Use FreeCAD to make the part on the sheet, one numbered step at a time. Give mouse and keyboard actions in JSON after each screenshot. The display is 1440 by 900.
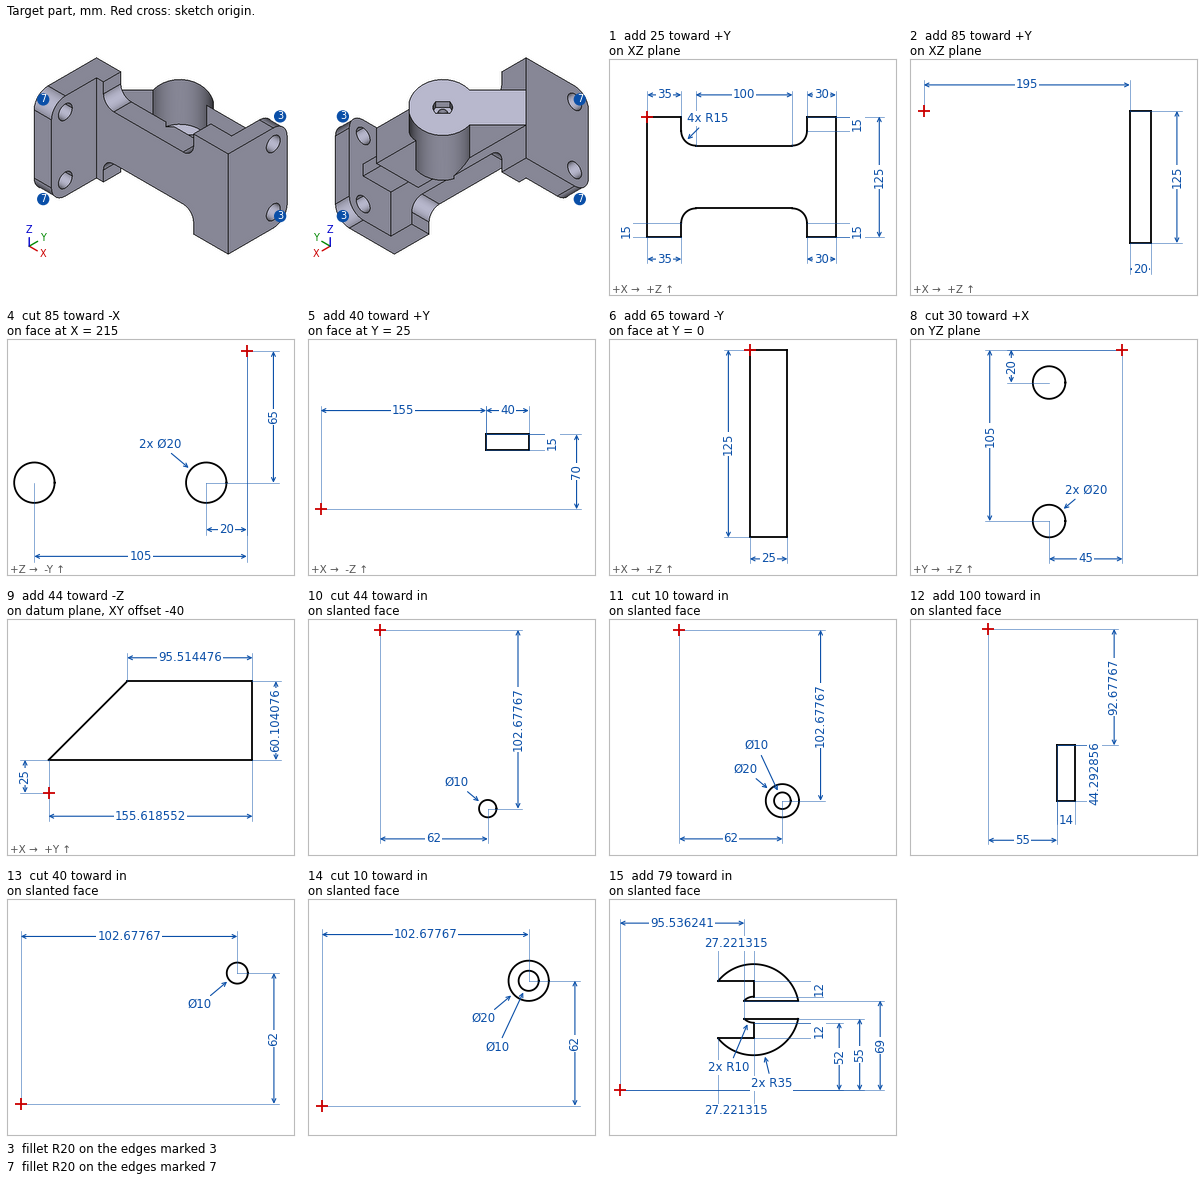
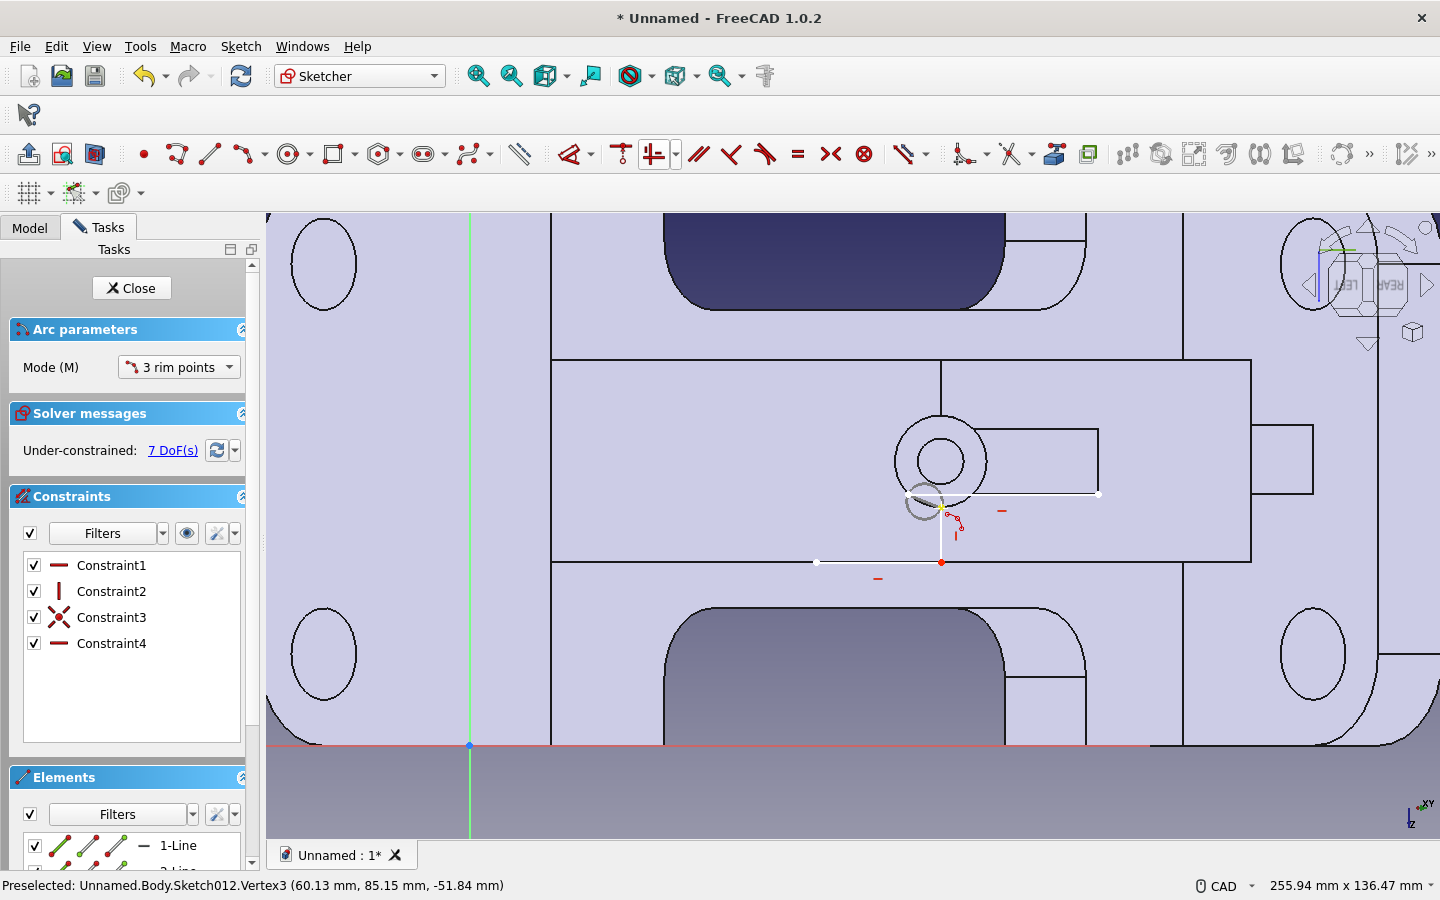
{"action": "scroll", "coordinate": [923, 504], "scroll_direction": "up", "scroll_amount": 8}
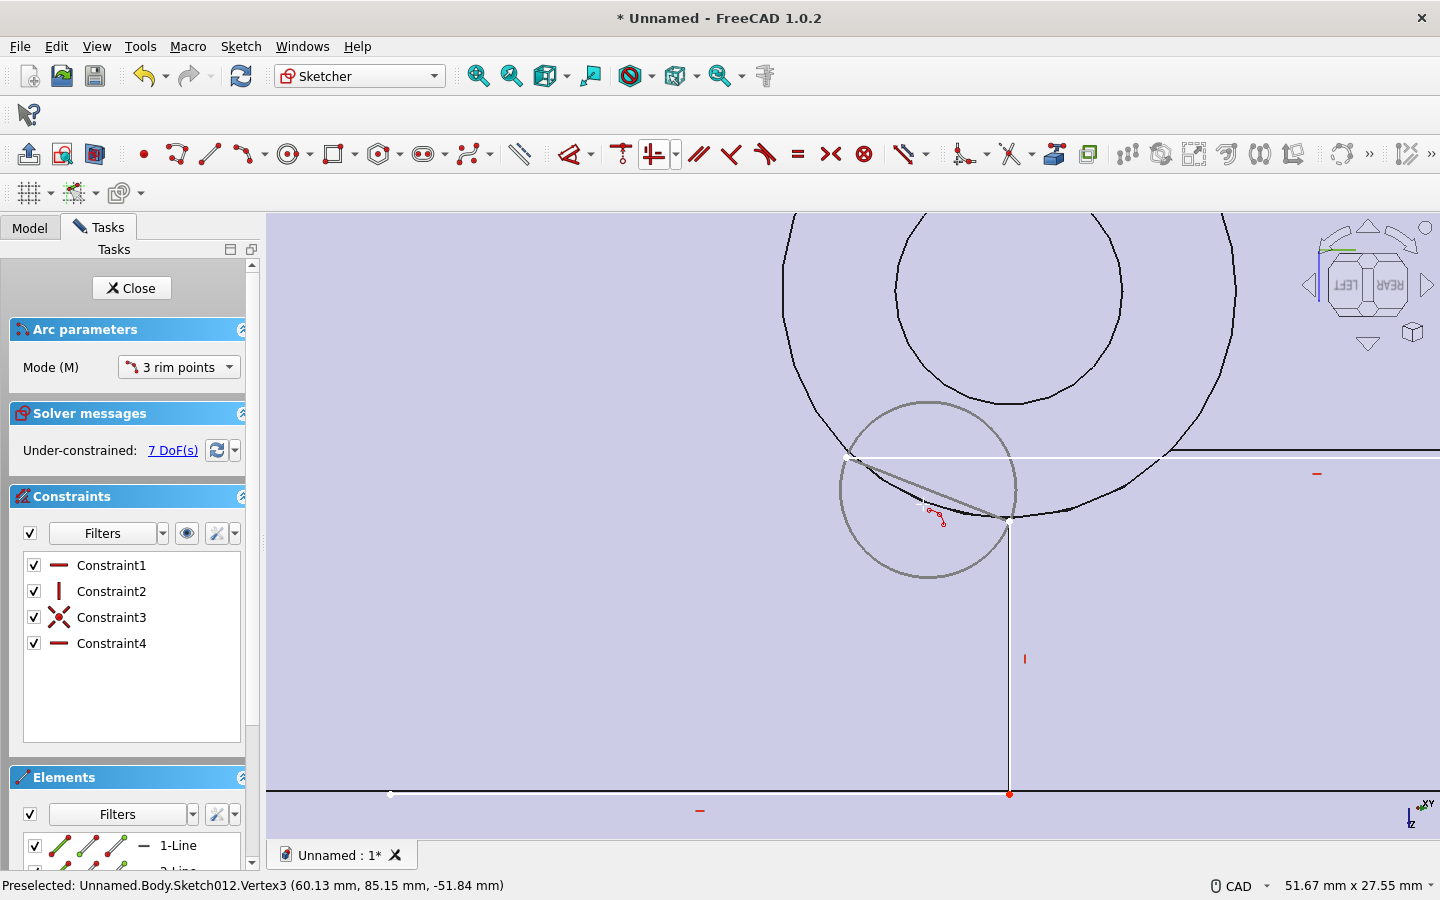
{"action": "left_click", "coordinate": [921, 501]}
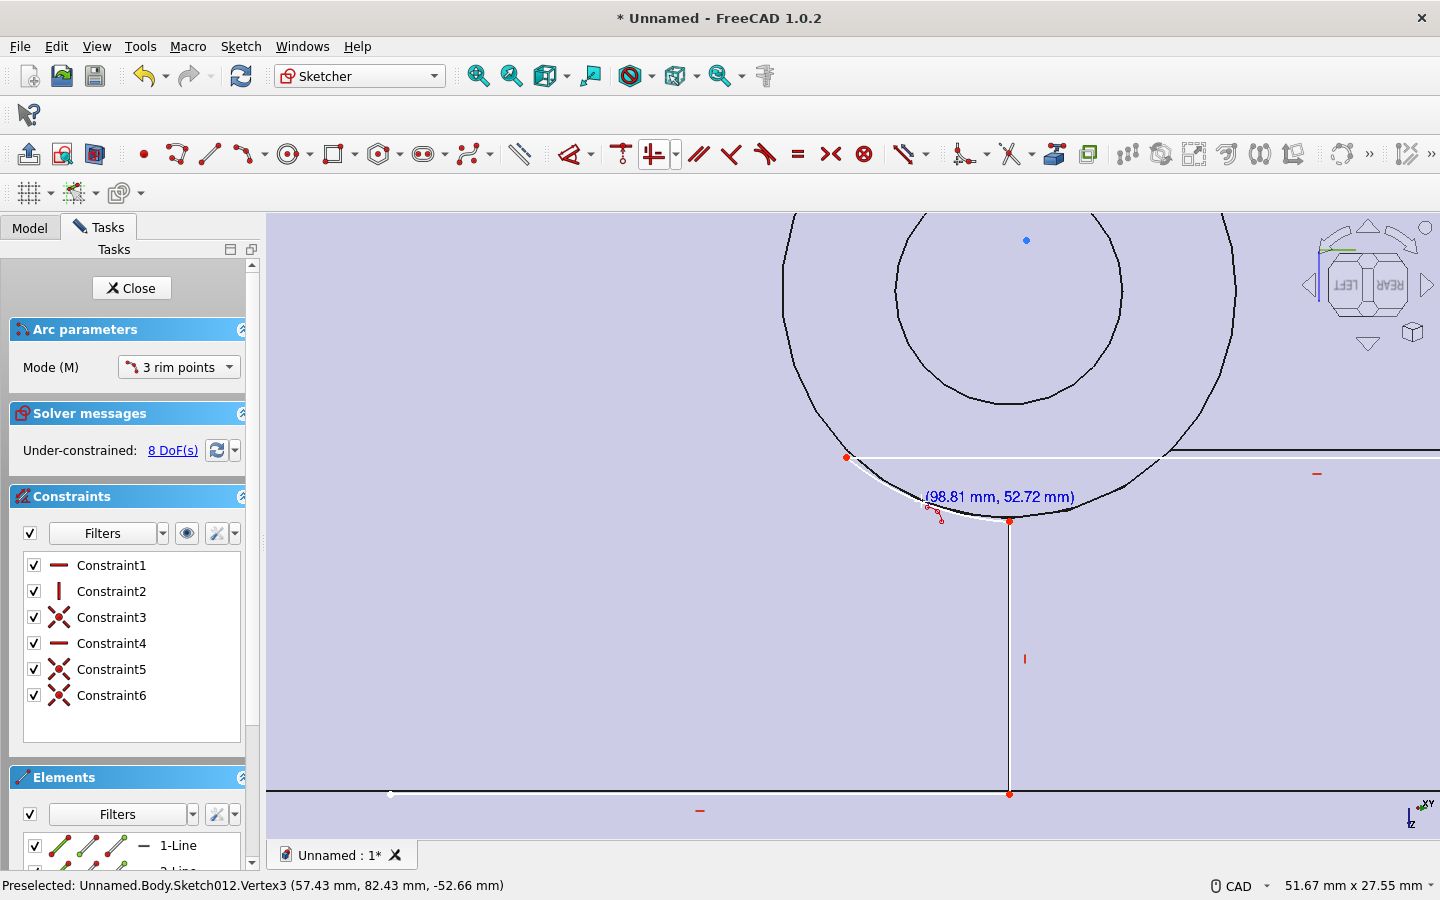
{"action": "scroll", "coordinate": [924, 505], "scroll_direction": "down", "scroll_amount": 8}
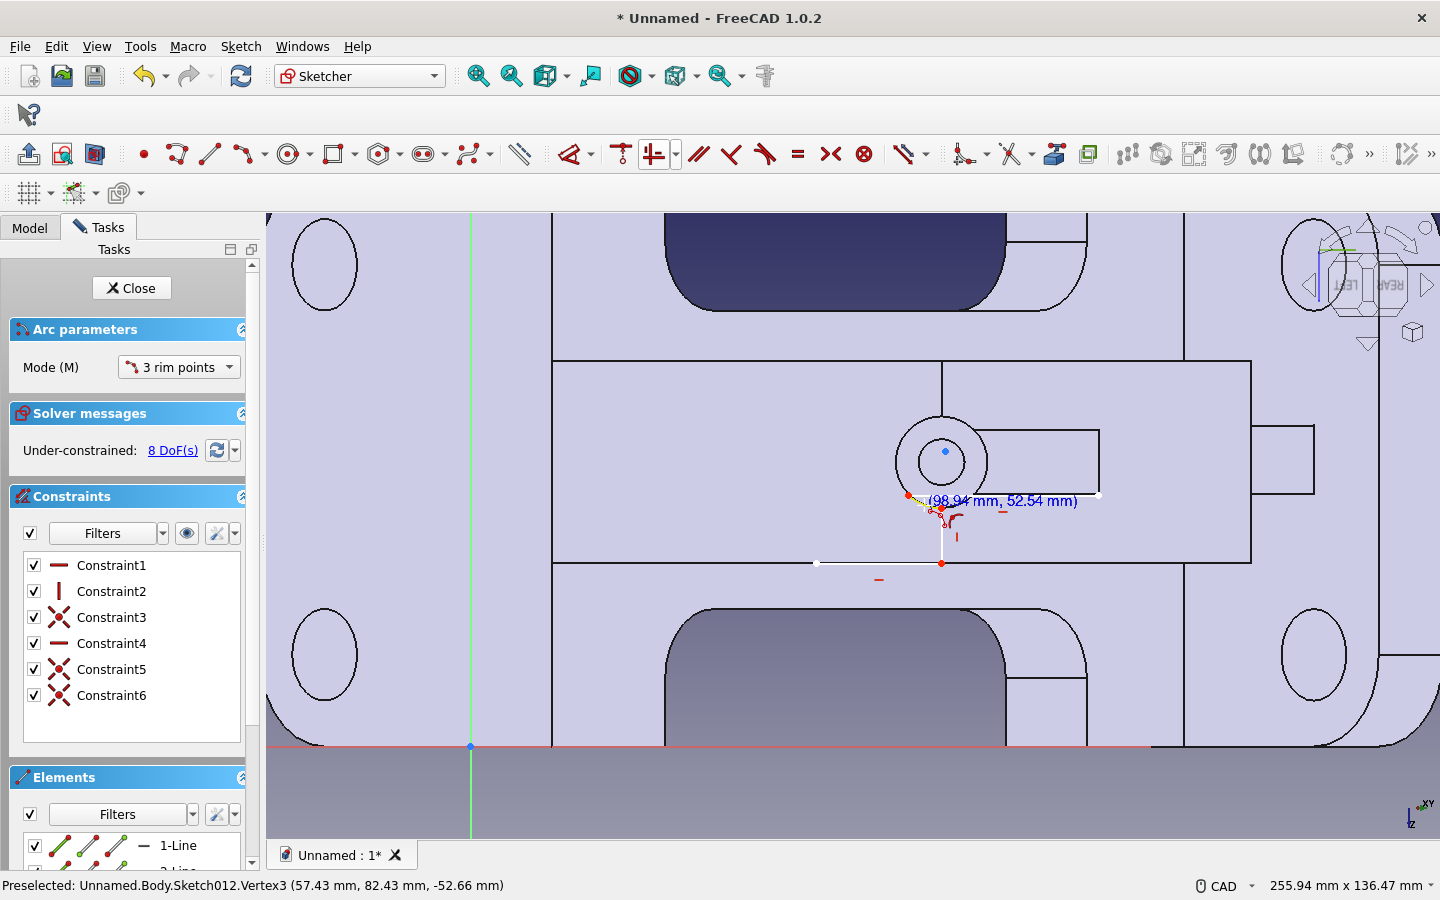
{"action": "left_click", "coordinate": [817, 564]}
{"action": "left_click", "coordinate": [1099, 496]}
{"action": "left_click", "coordinate": [980, 618]}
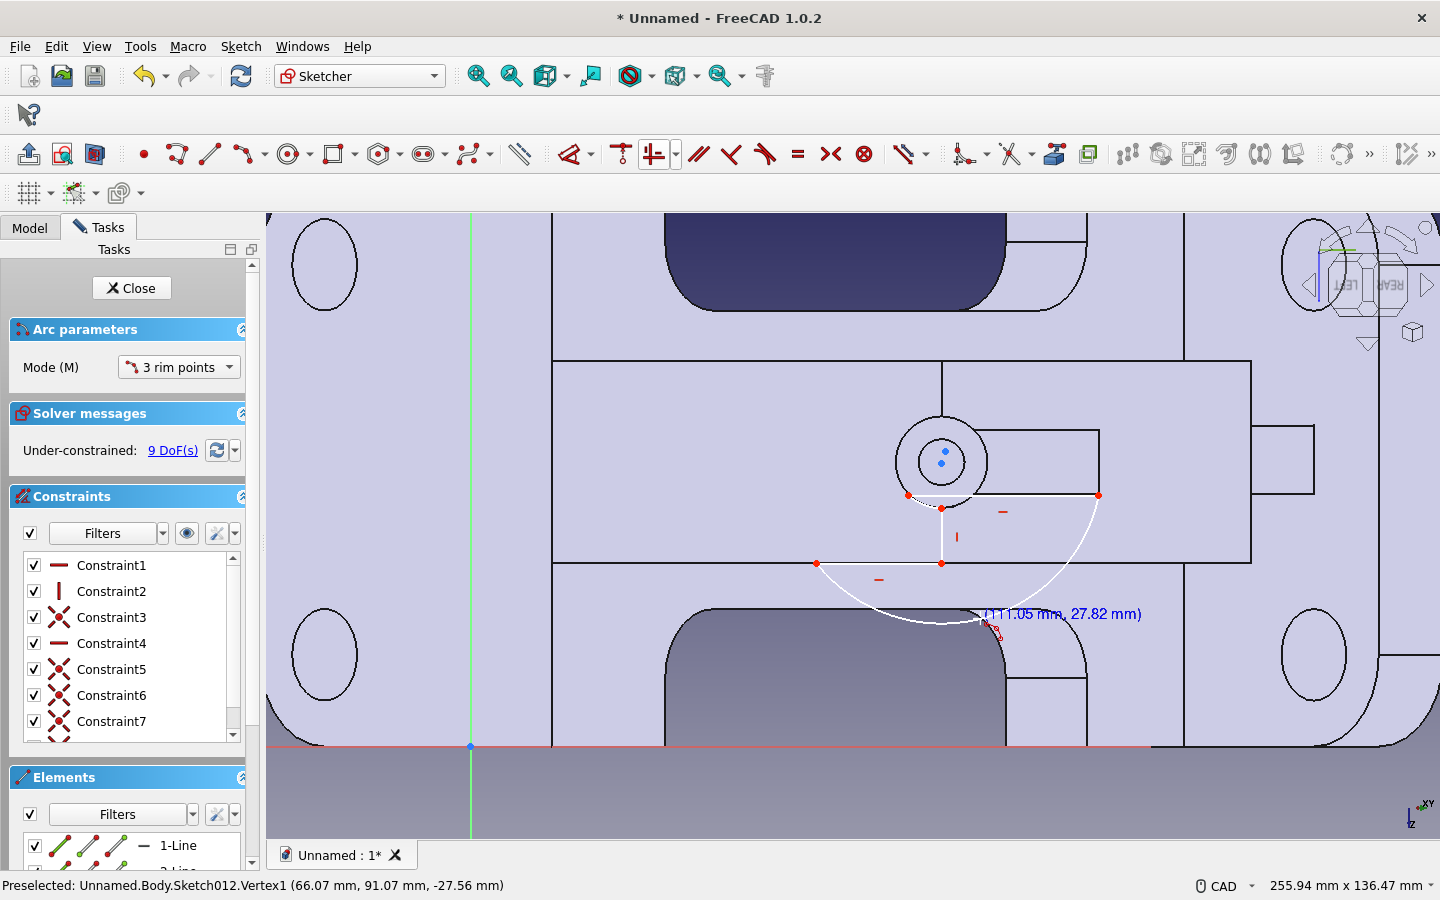
{"action": "left_click", "coordinate": [210, 154]}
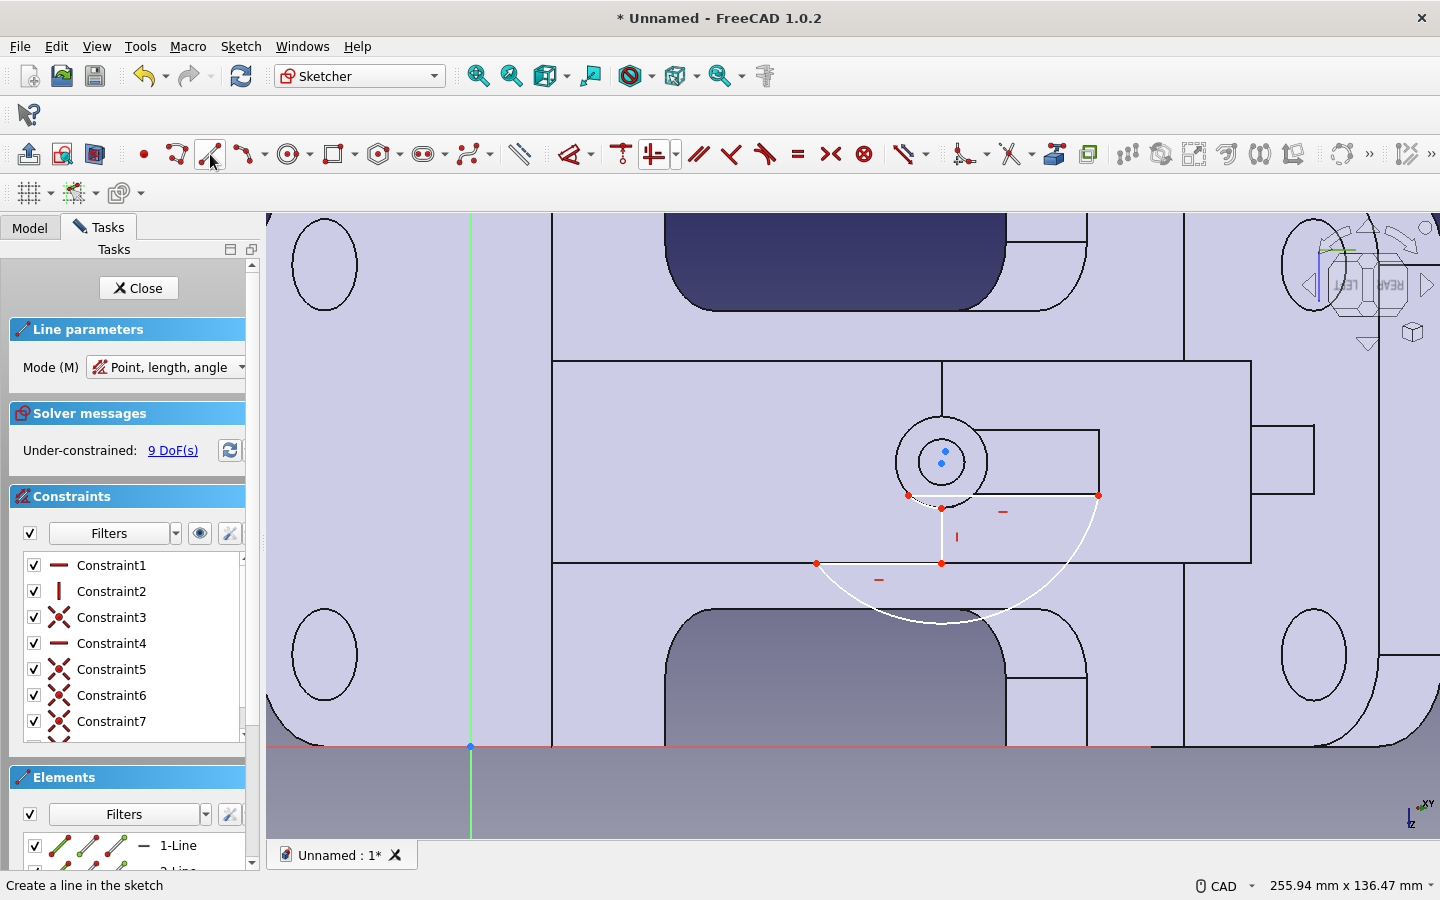
{"action": "left_click", "coordinate": [909, 430]}
{"action": "left_click", "coordinate": [1099, 430]}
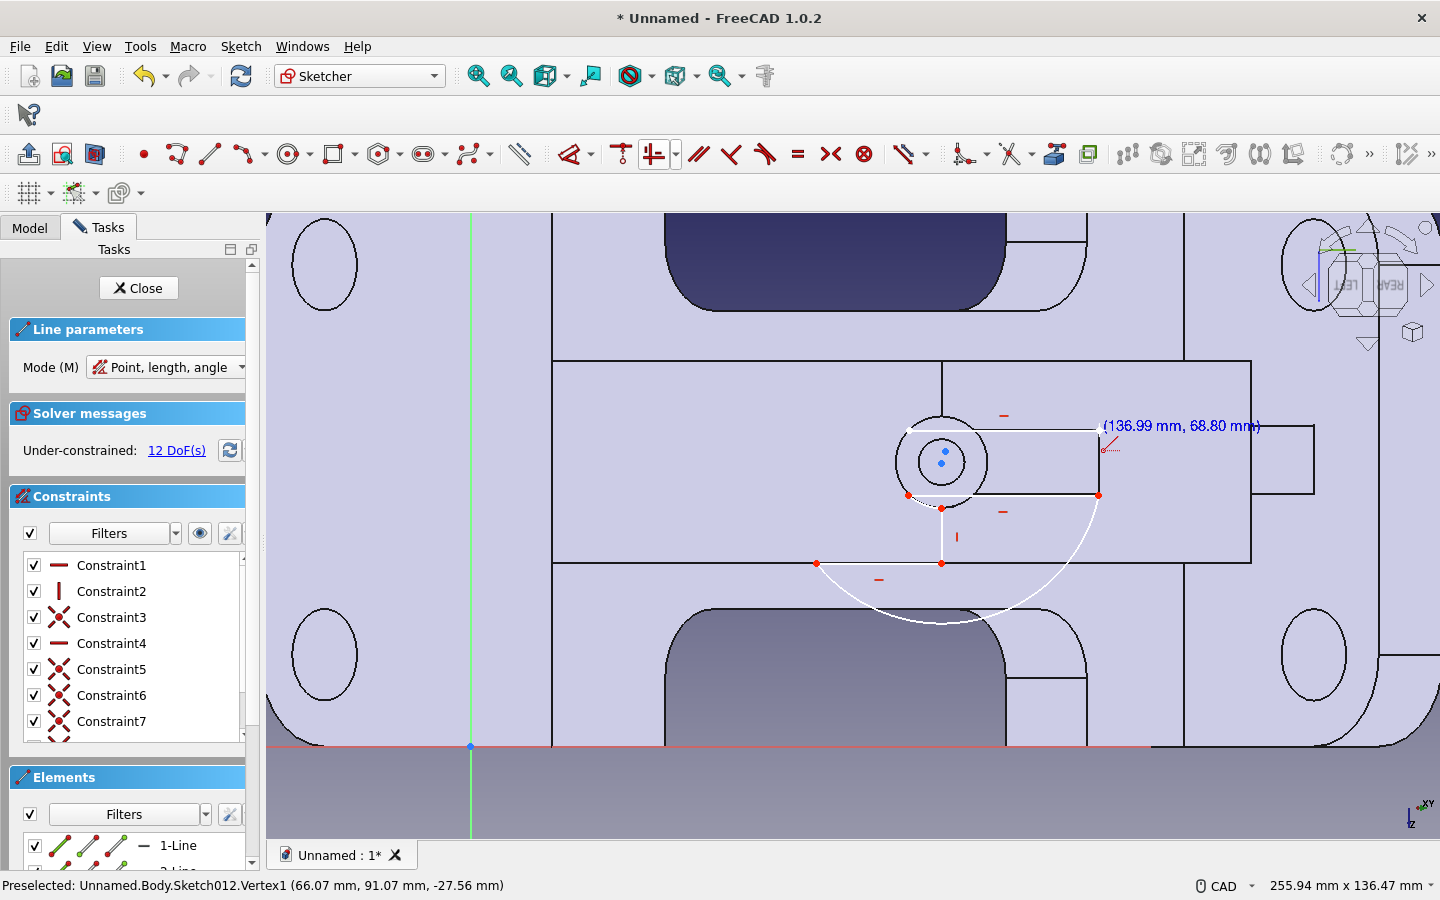
{"action": "left_click", "coordinate": [177, 154]}